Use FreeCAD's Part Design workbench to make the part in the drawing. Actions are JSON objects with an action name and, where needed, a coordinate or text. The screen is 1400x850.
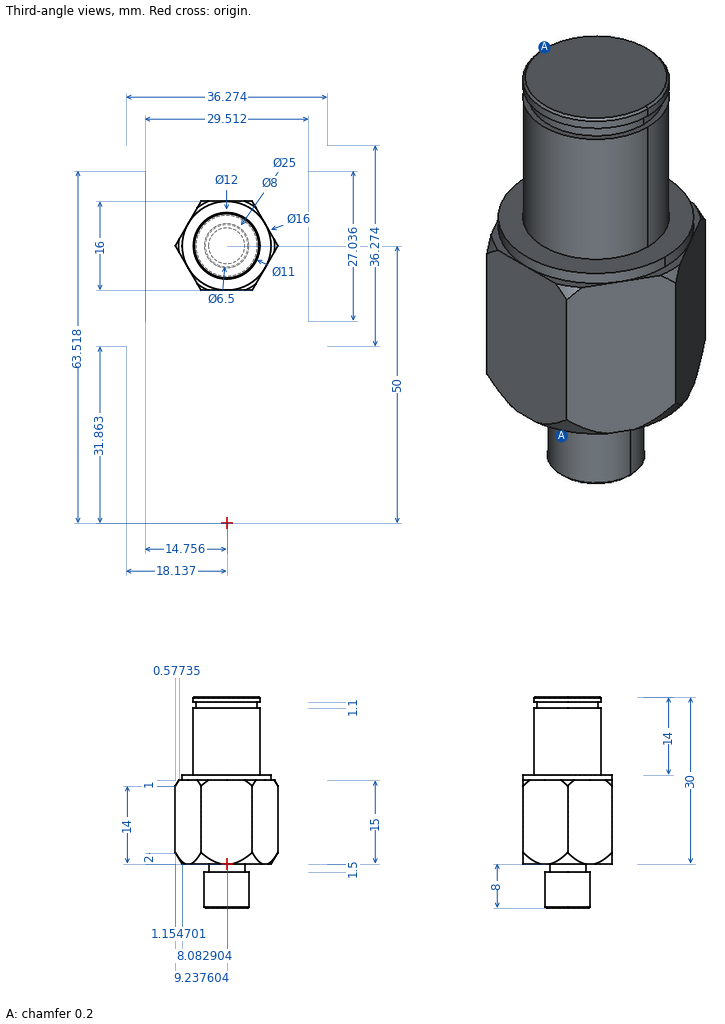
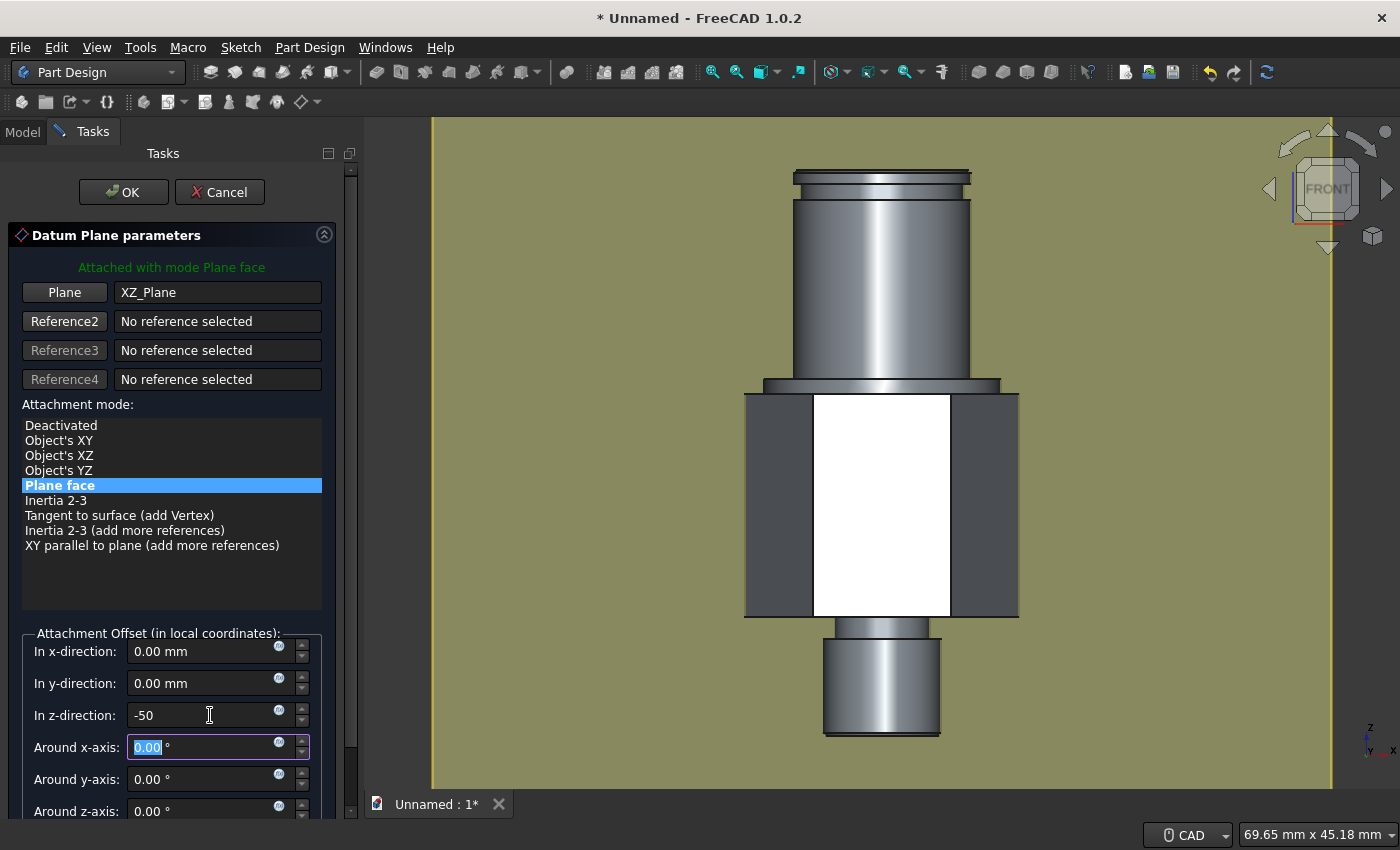
{"action": "left_click", "coordinate": [124, 192]}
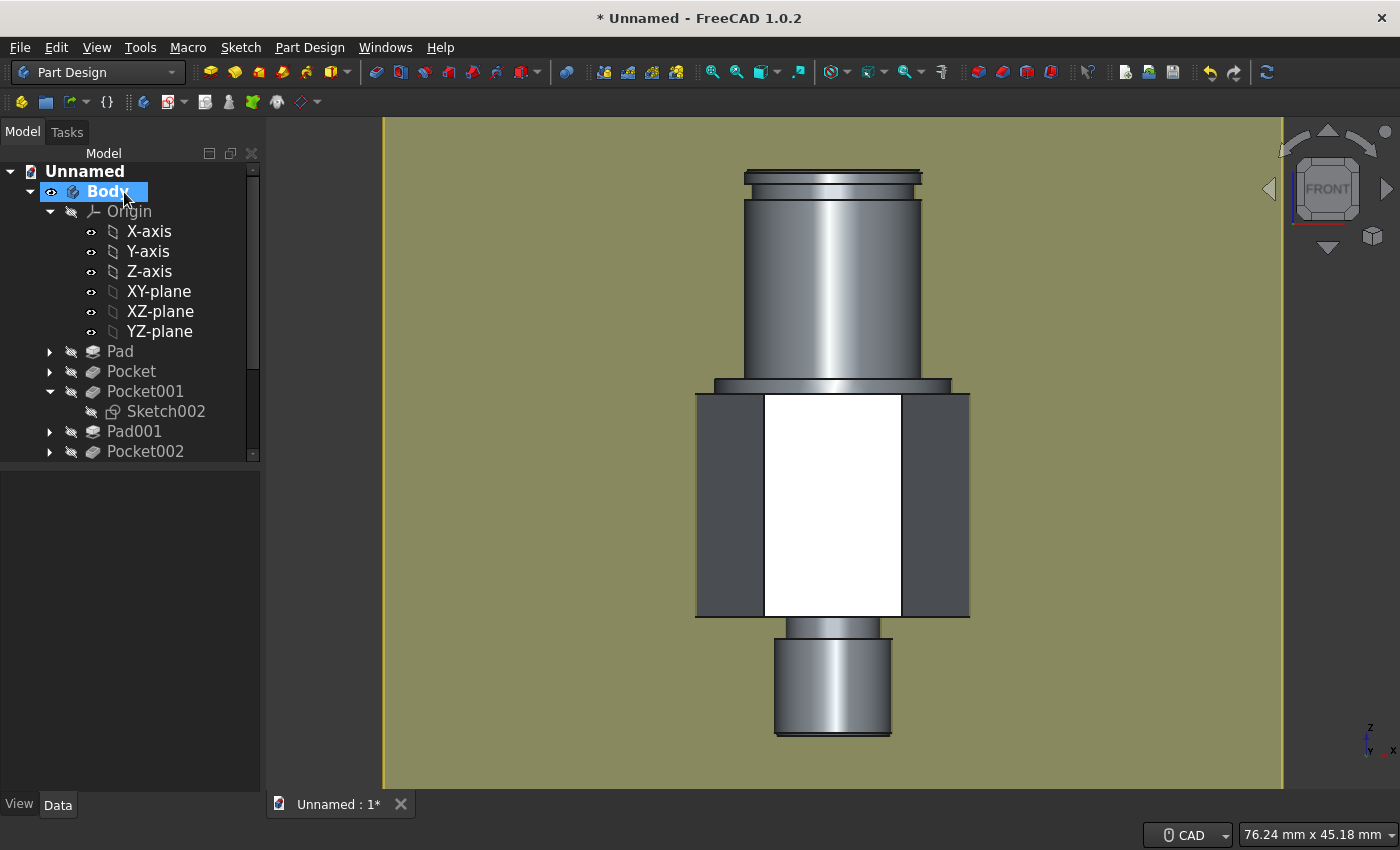
{"action": "scroll", "coordinate": [100, 307], "scroll_direction": "down", "scroll_amount": 3}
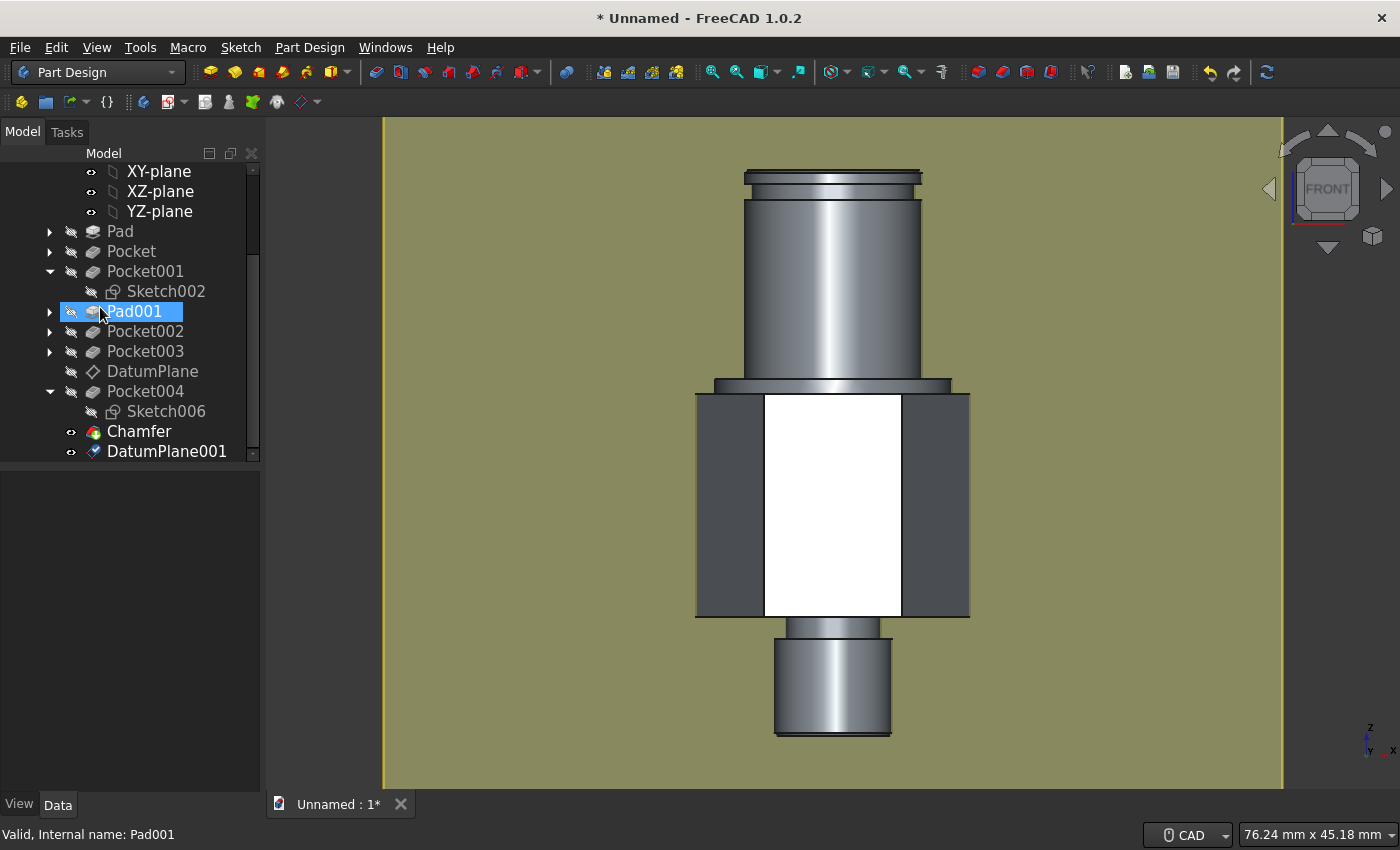
{"action": "left_click", "coordinate": [116, 452]}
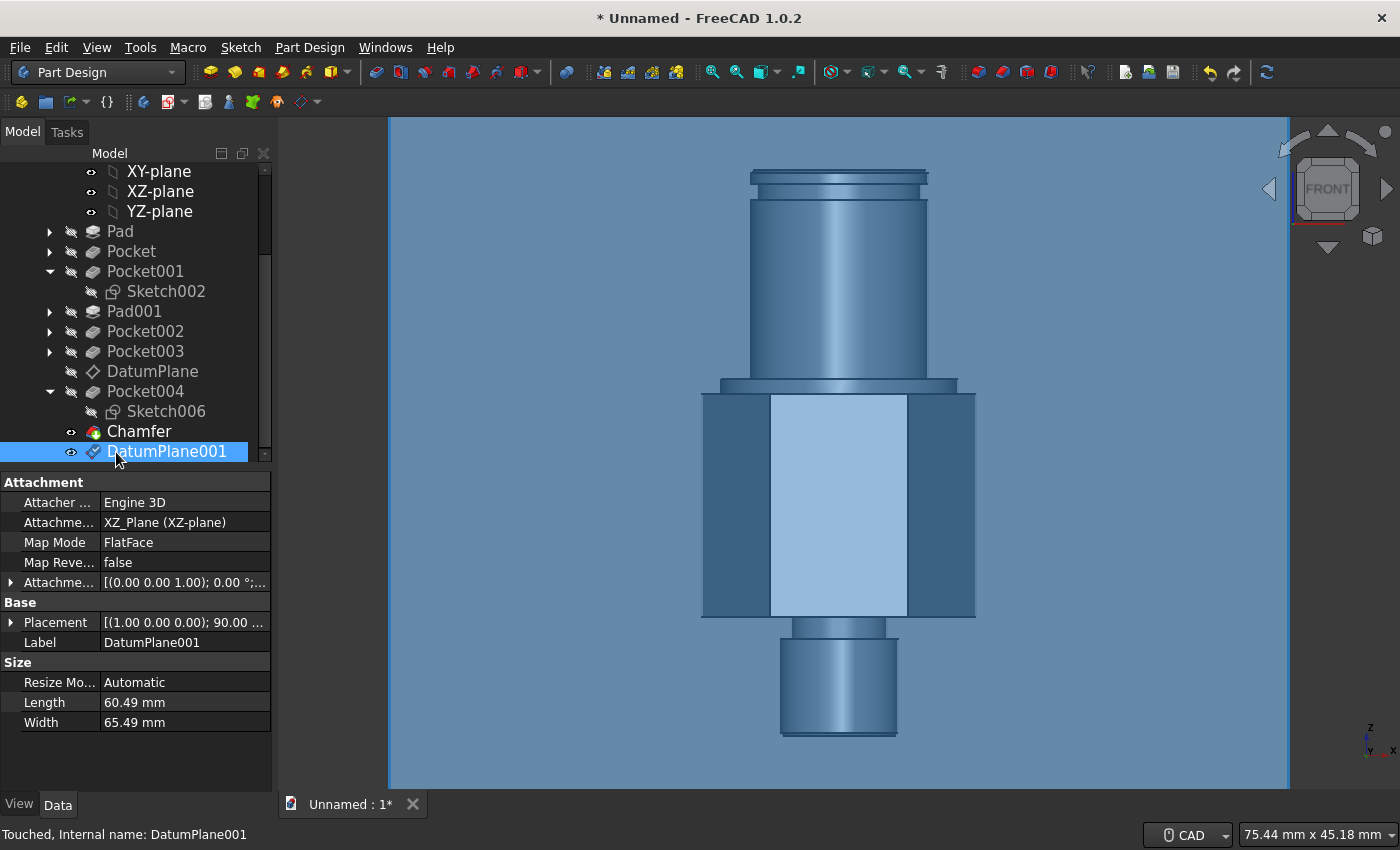
{"action": "left_click", "coordinate": [168, 102]}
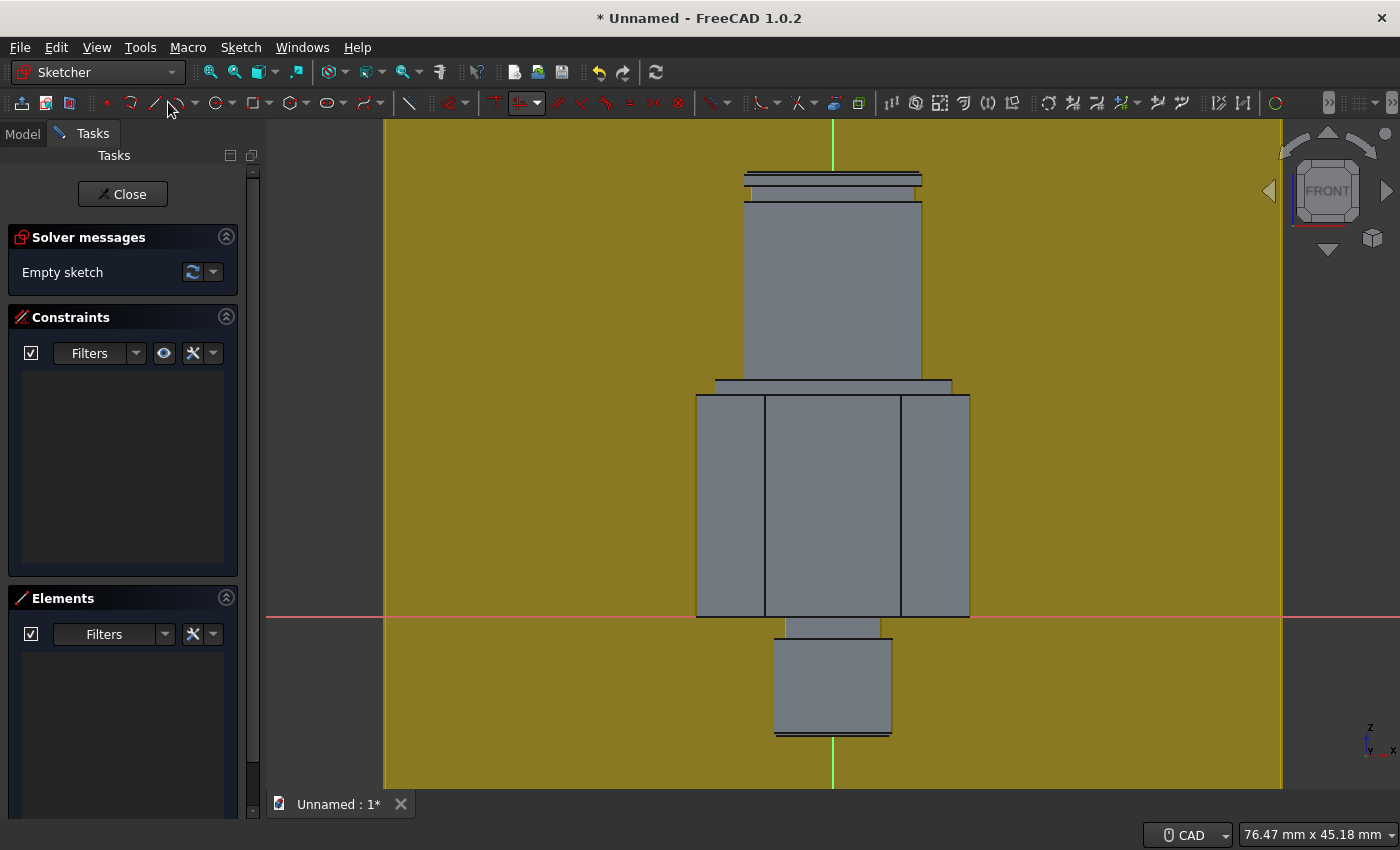
{"action": "left_click", "coordinate": [70, 104]}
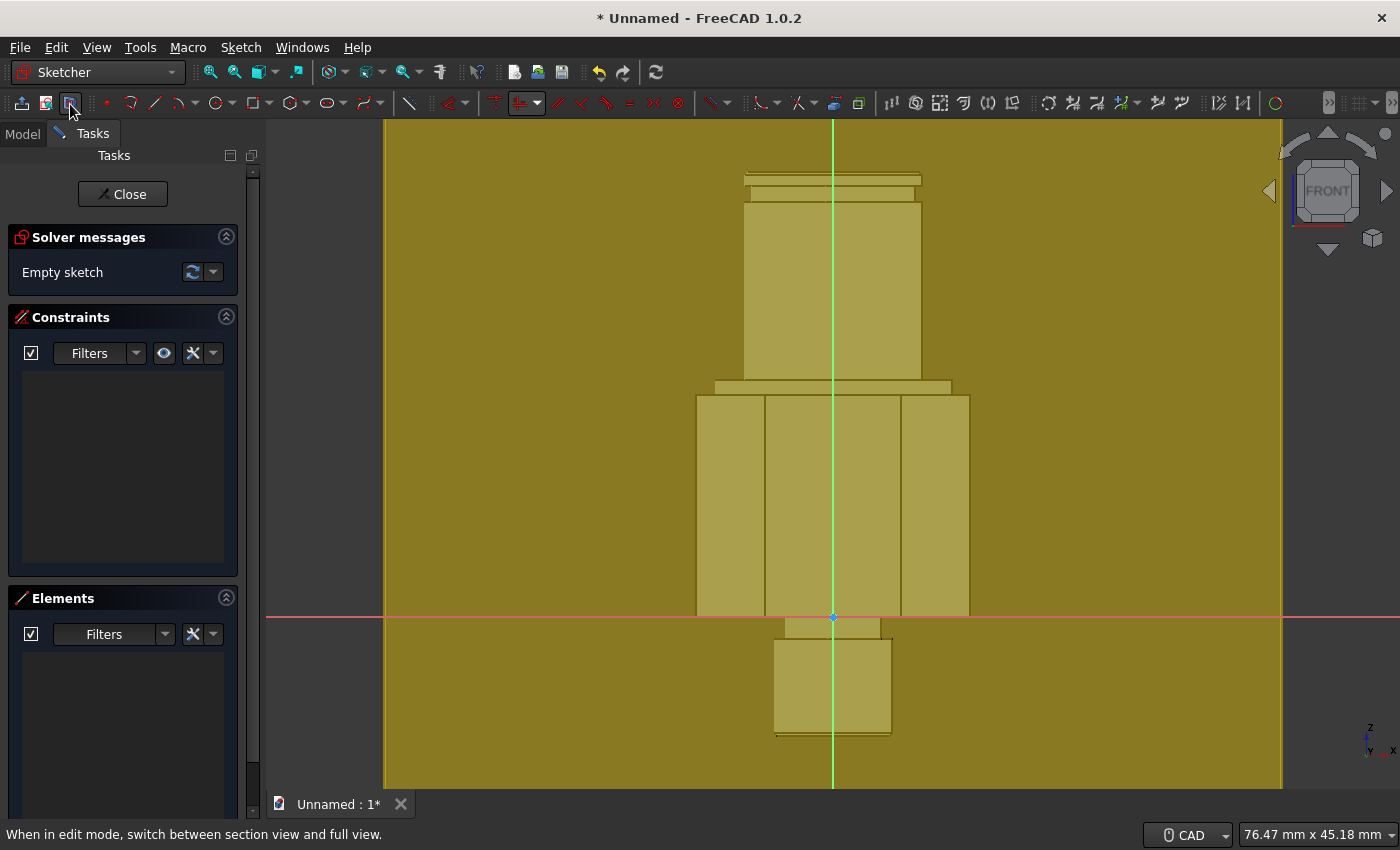
{"action": "scroll", "coordinate": [765, 569], "scroll_direction": "up", "scroll_amount": 3}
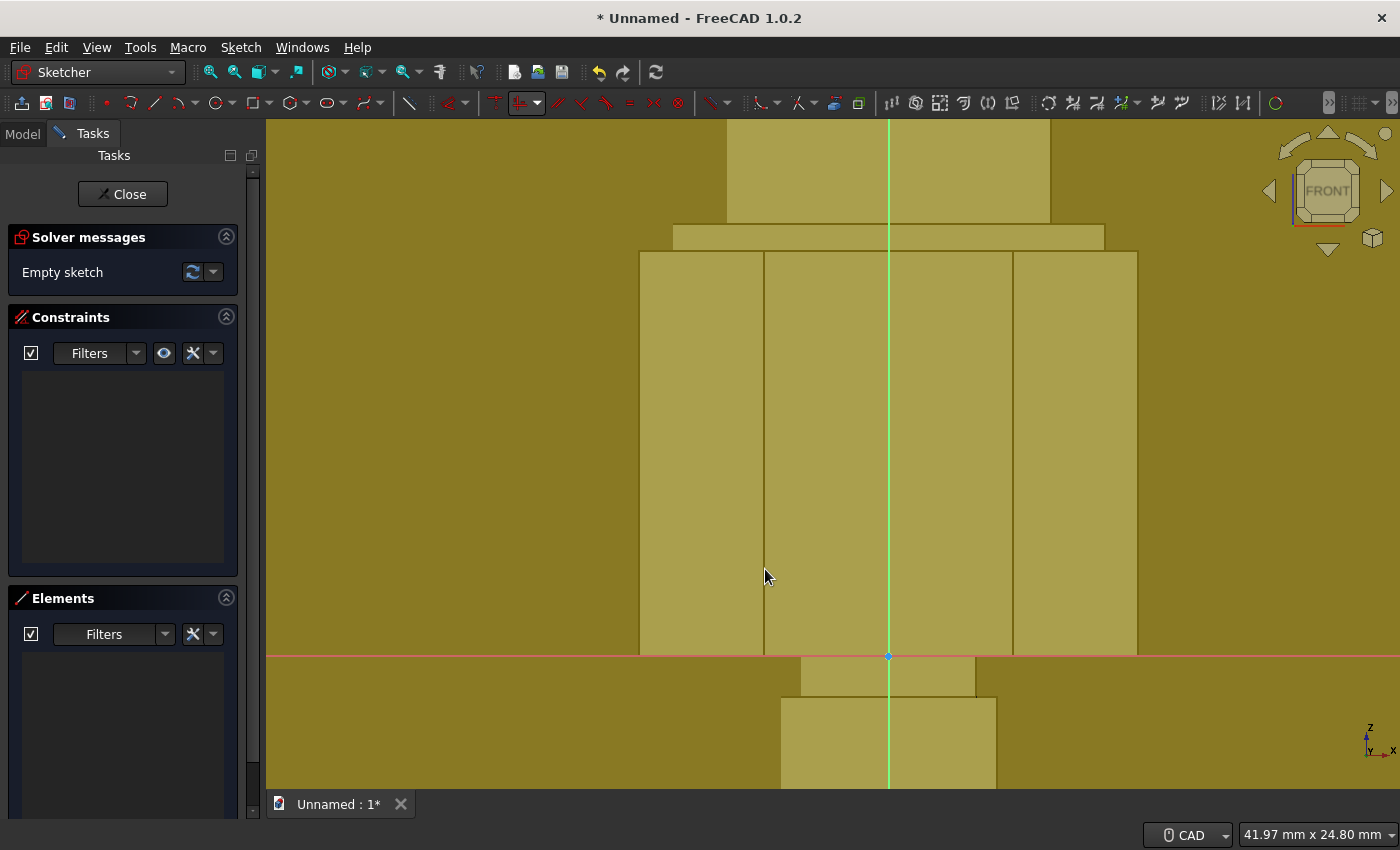
{"action": "left_click", "coordinate": [132, 104]}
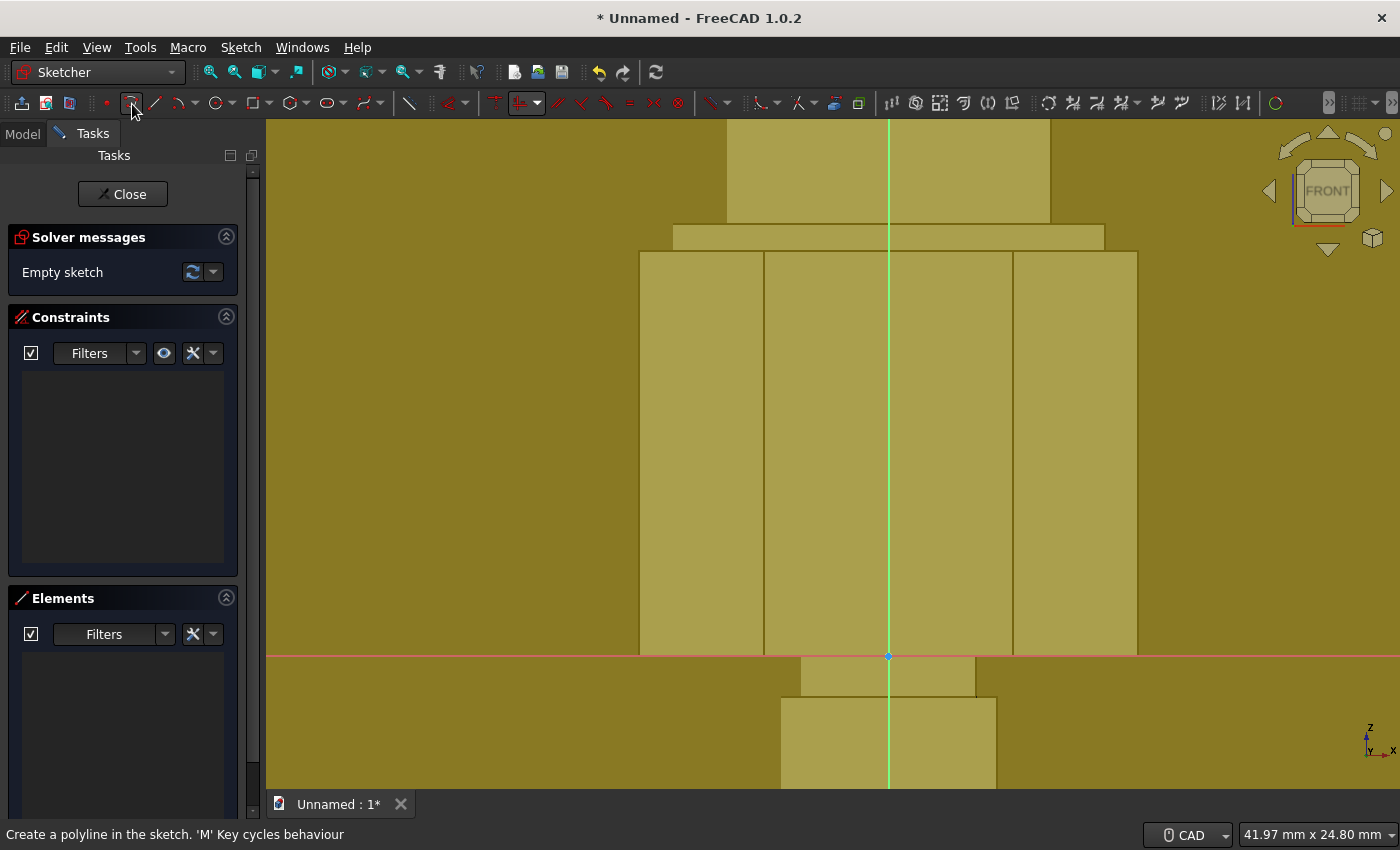
{"action": "left_click", "coordinate": [670, 656]}
{"action": "left_click", "coordinate": [639, 647]}
{"action": "left_click", "coordinate": [639, 602]}
{"action": "left_click", "coordinate": [670, 656]}